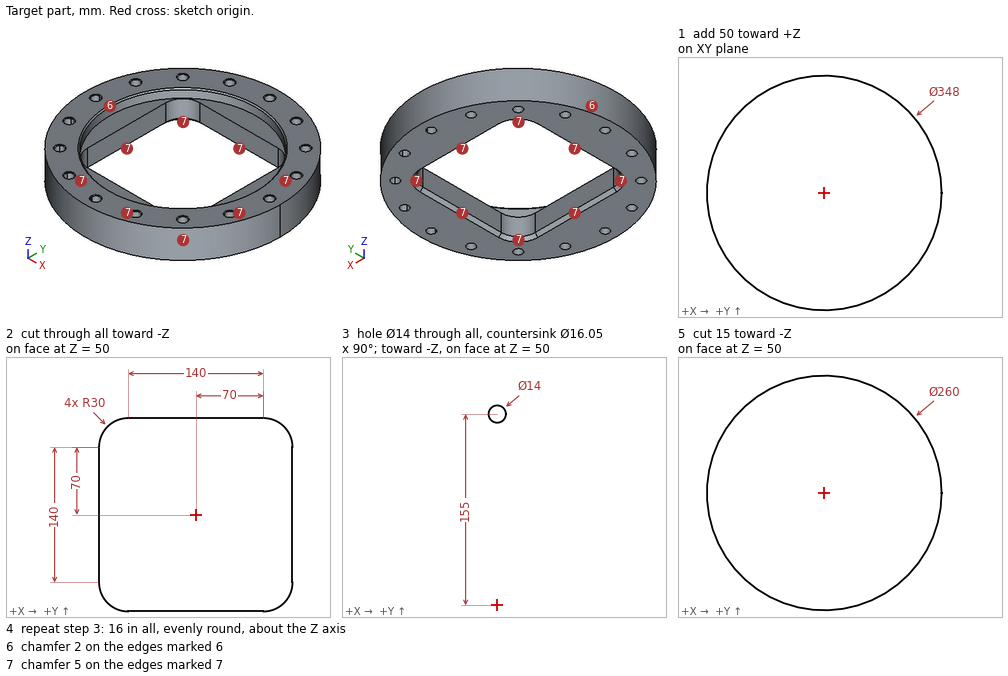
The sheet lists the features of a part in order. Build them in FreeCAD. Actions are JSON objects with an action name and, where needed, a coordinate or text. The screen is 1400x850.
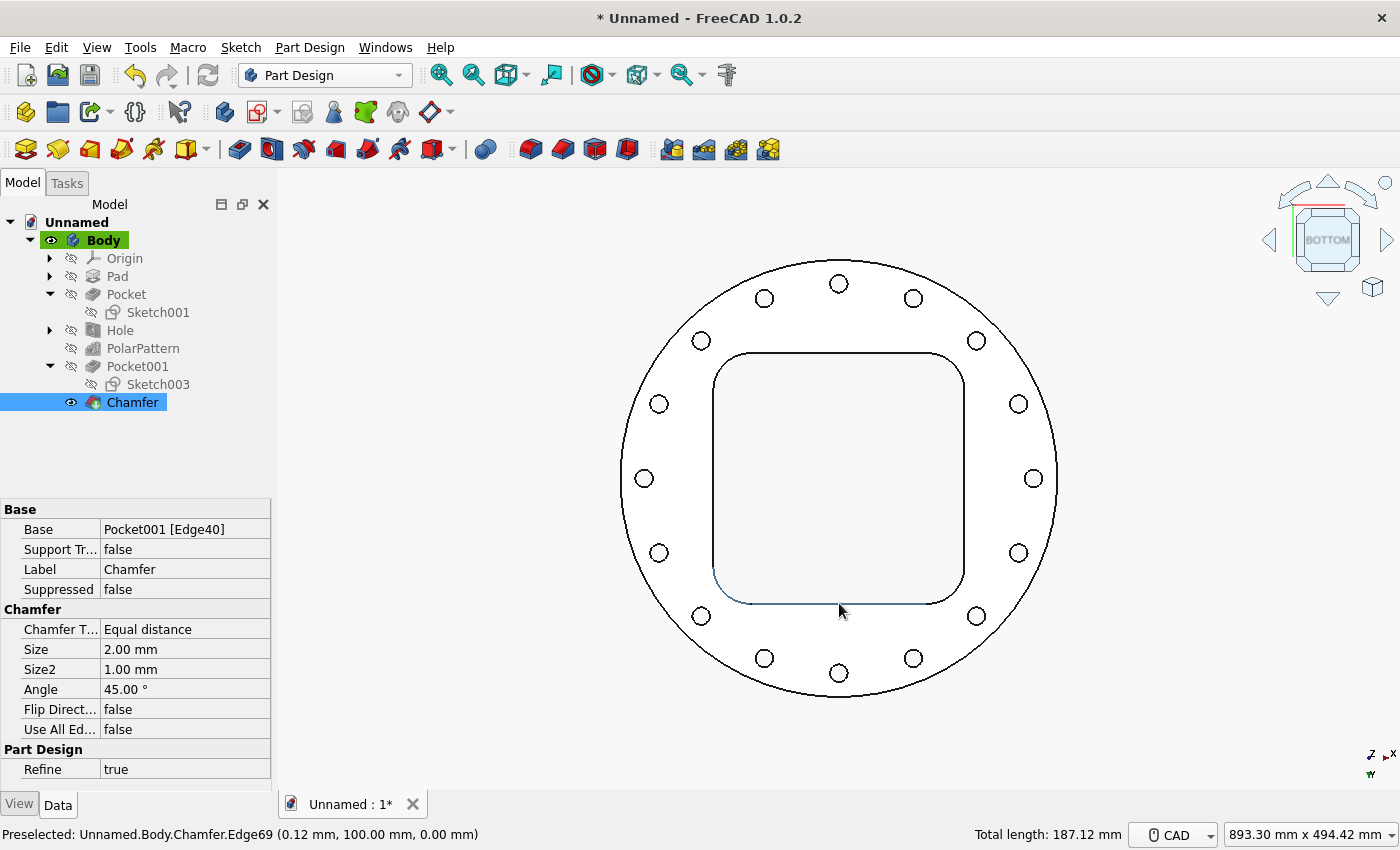
{"action": "left_click", "coordinate": [953, 592], "text": "ctrl"}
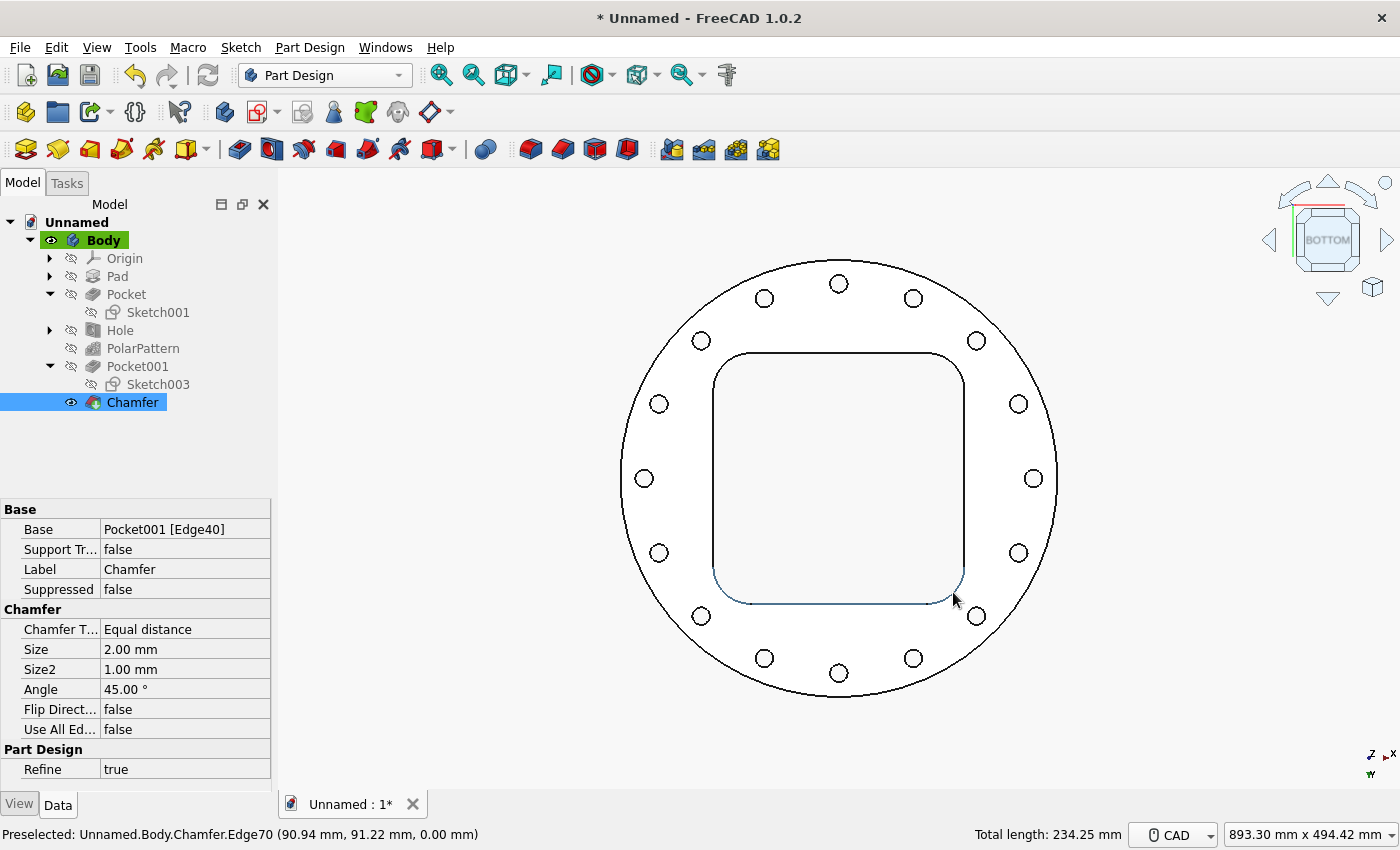
{"action": "left_click", "coordinate": [964, 477], "text": "ctrl"}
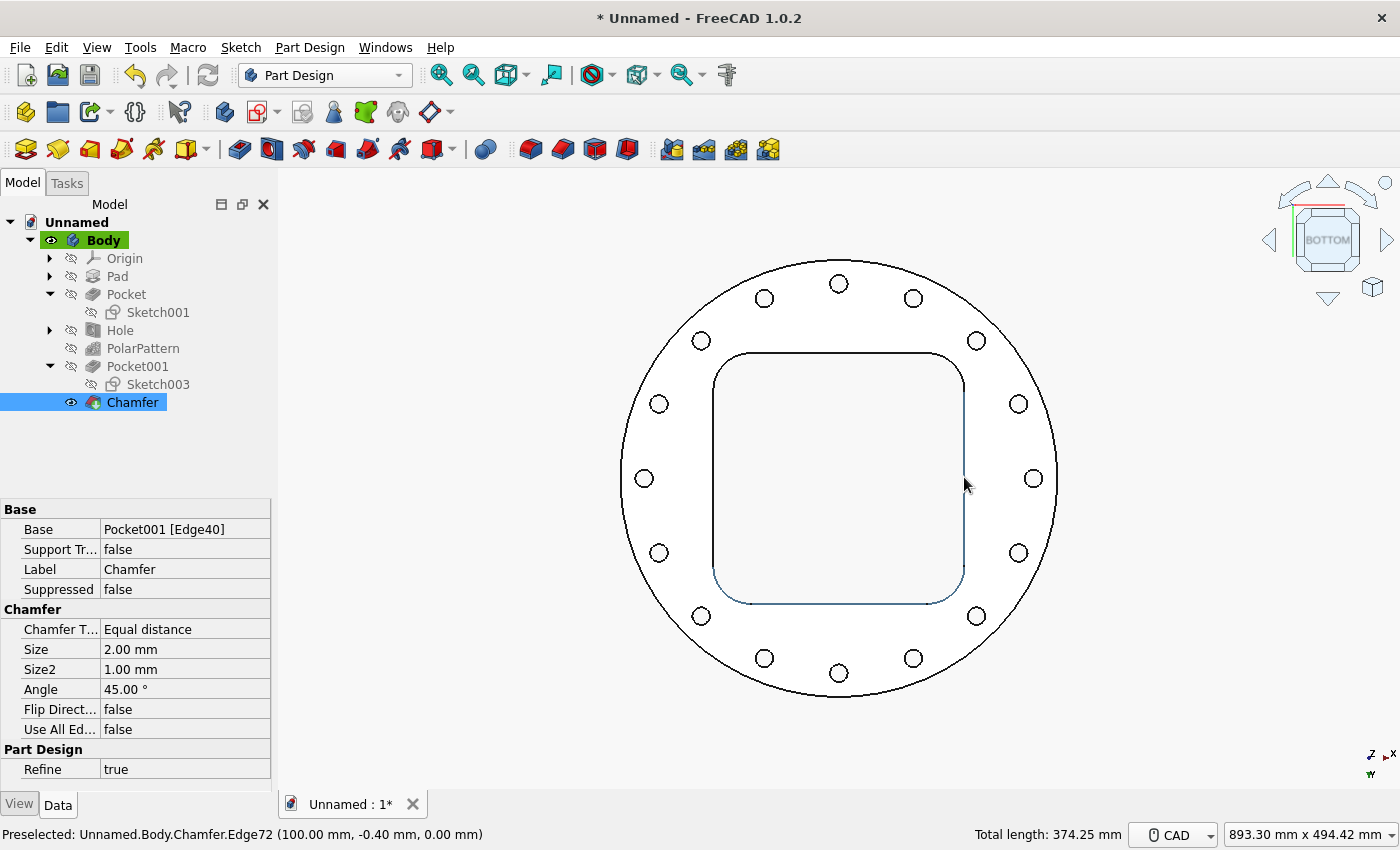
{"action": "left_click", "coordinate": [949, 359], "text": "ctrl"}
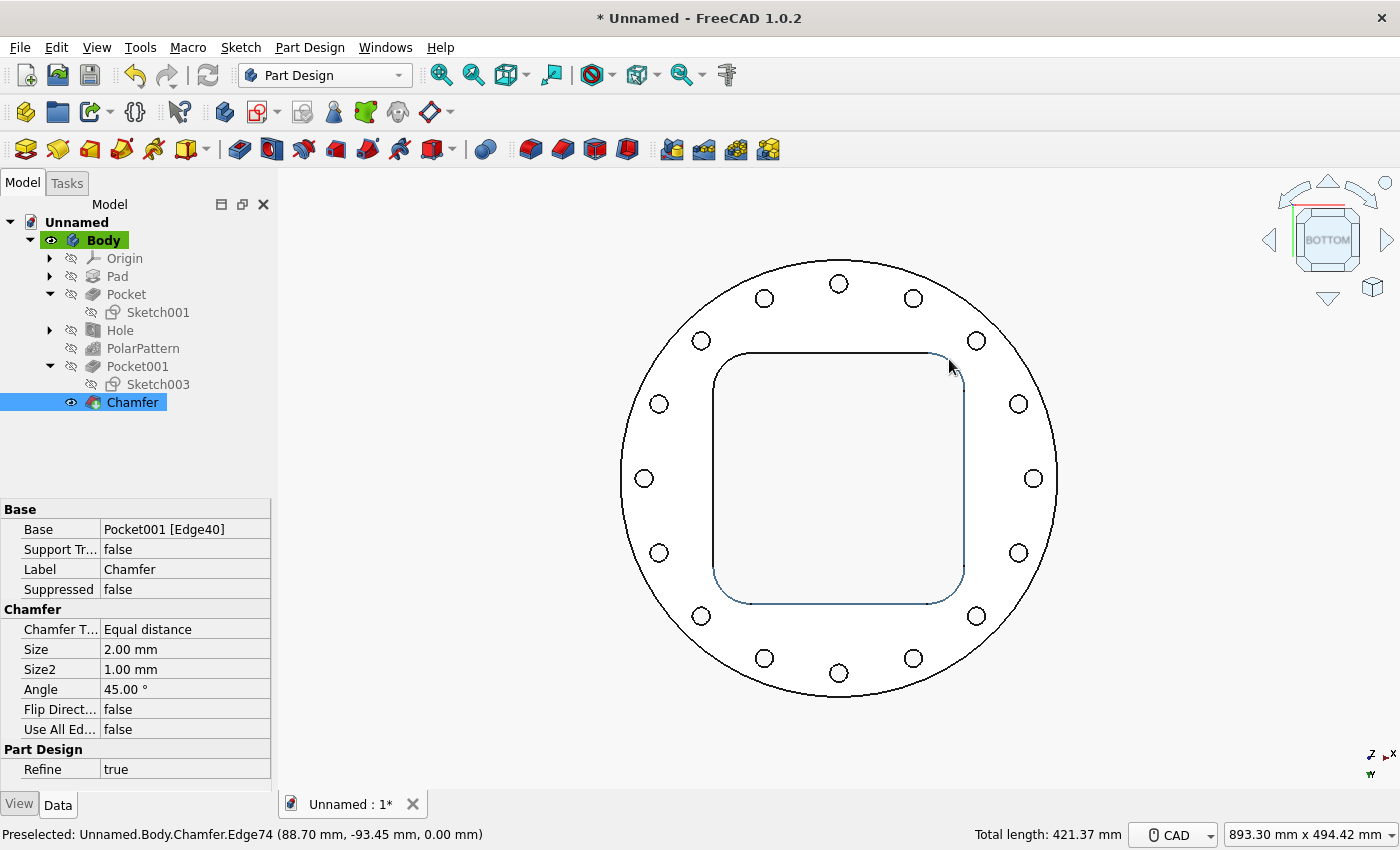
{"action": "key", "text": "4"}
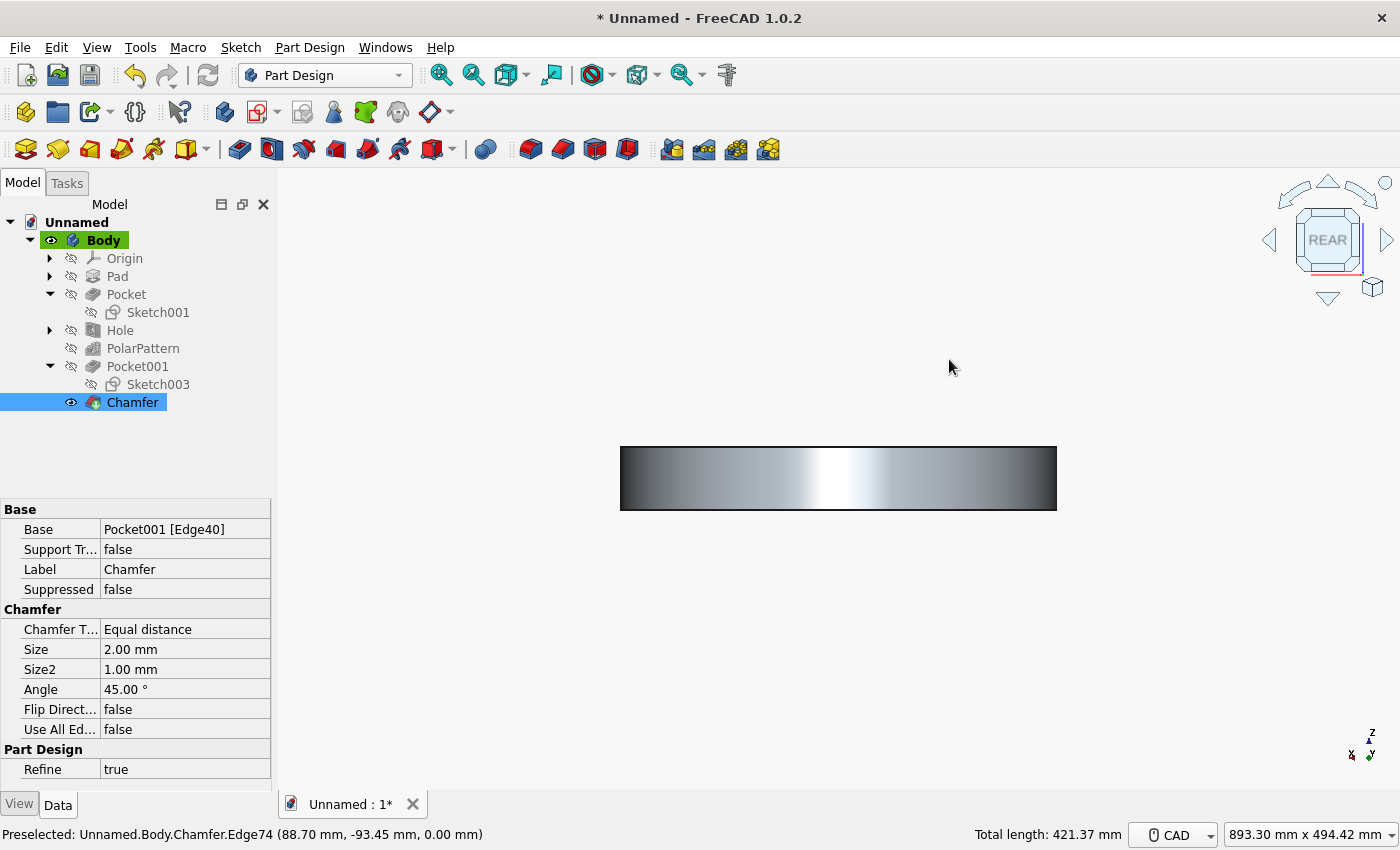
{"action": "left_click", "coordinate": [442, 76]}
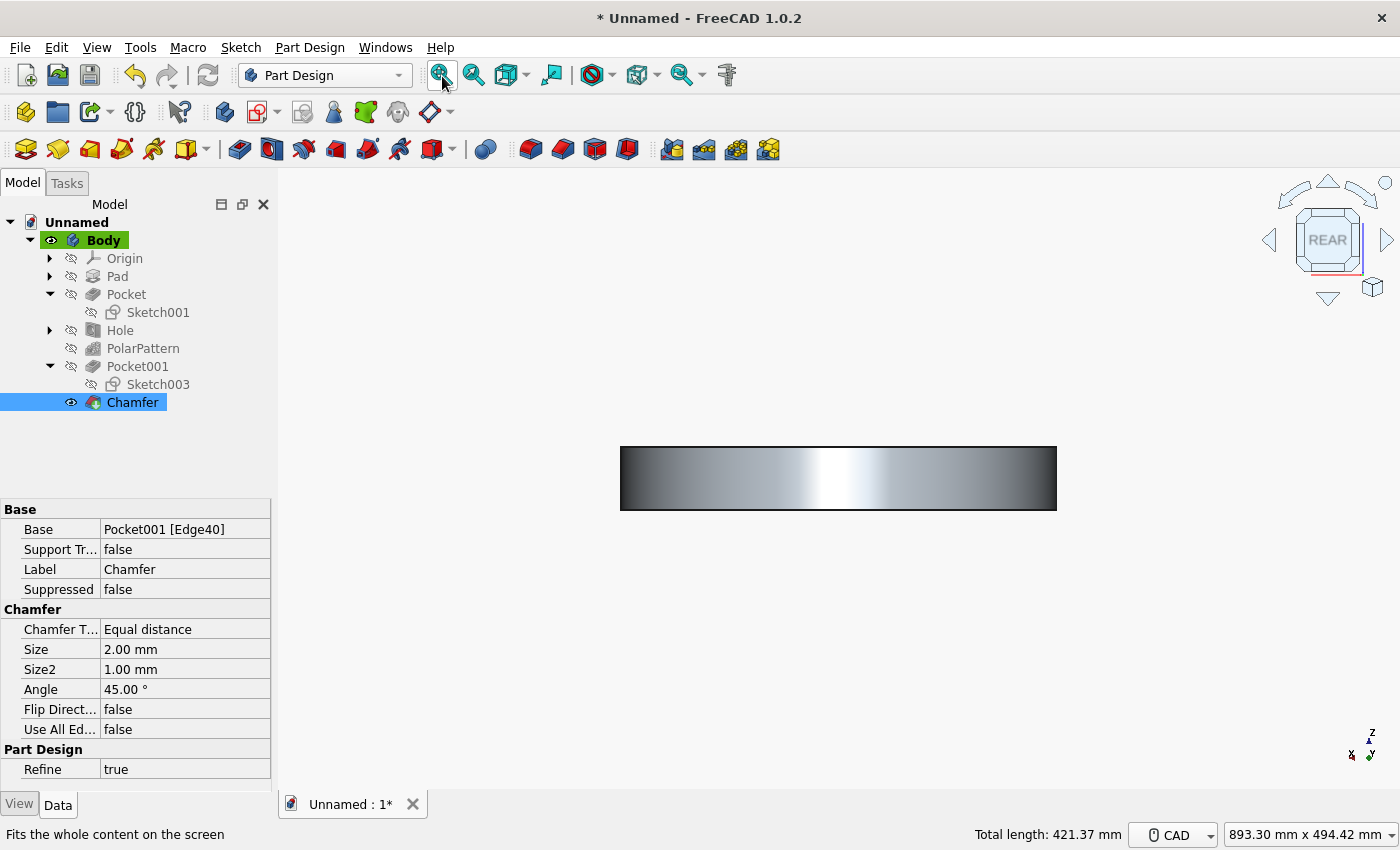
{"action": "key", "text": "6"}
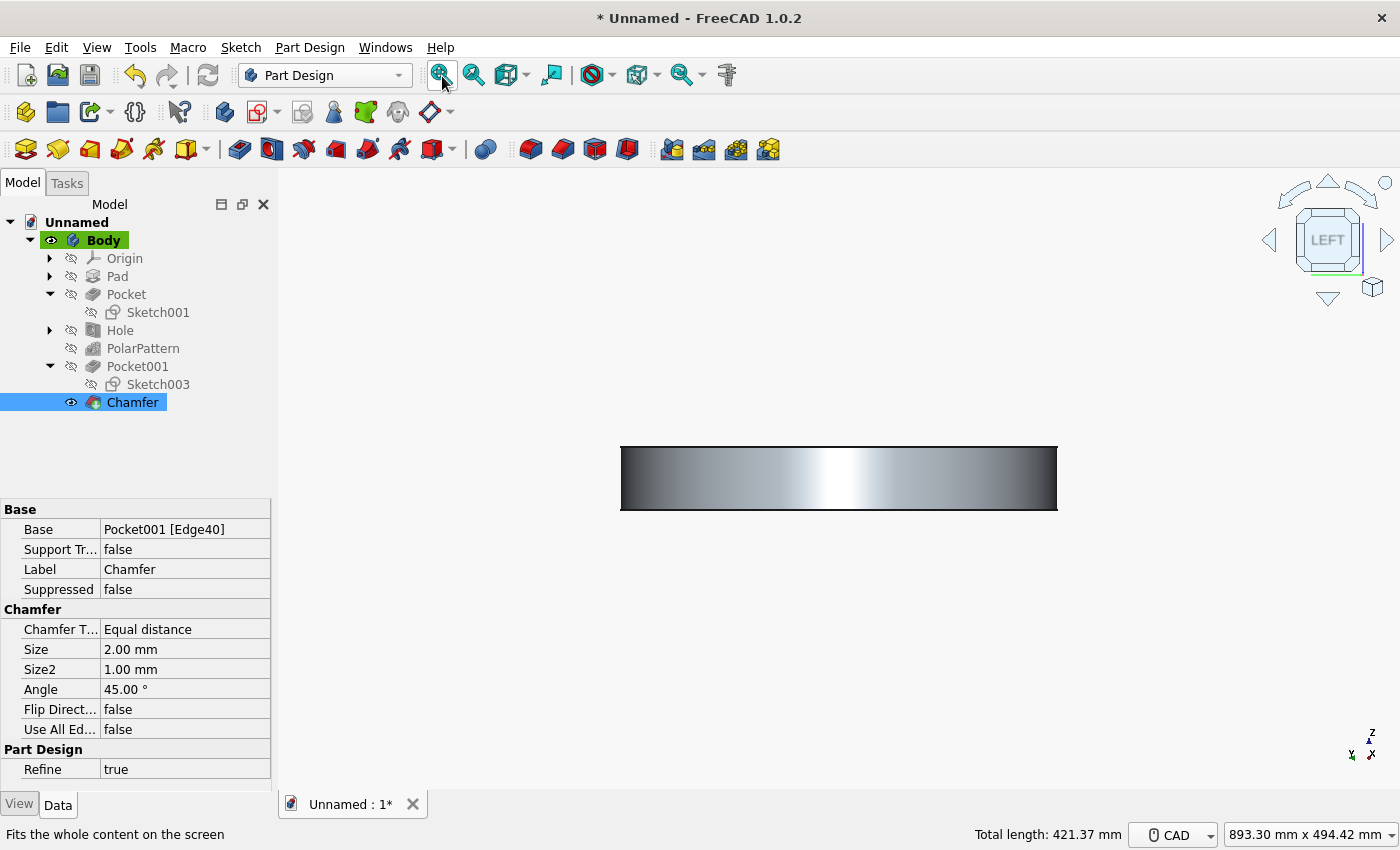
{"action": "left_click", "coordinate": [442, 76]}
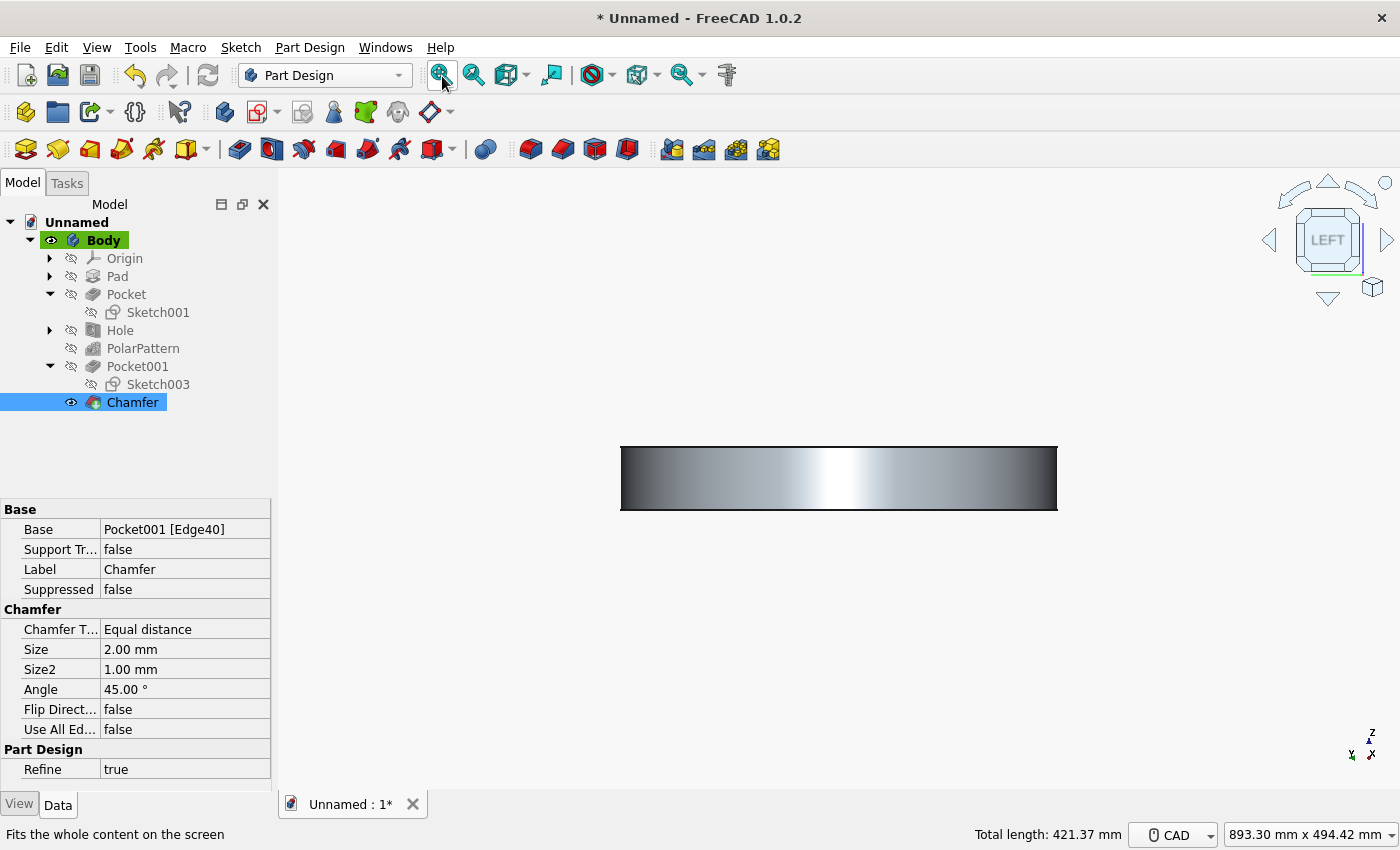
{"action": "key", "text": "v 3"}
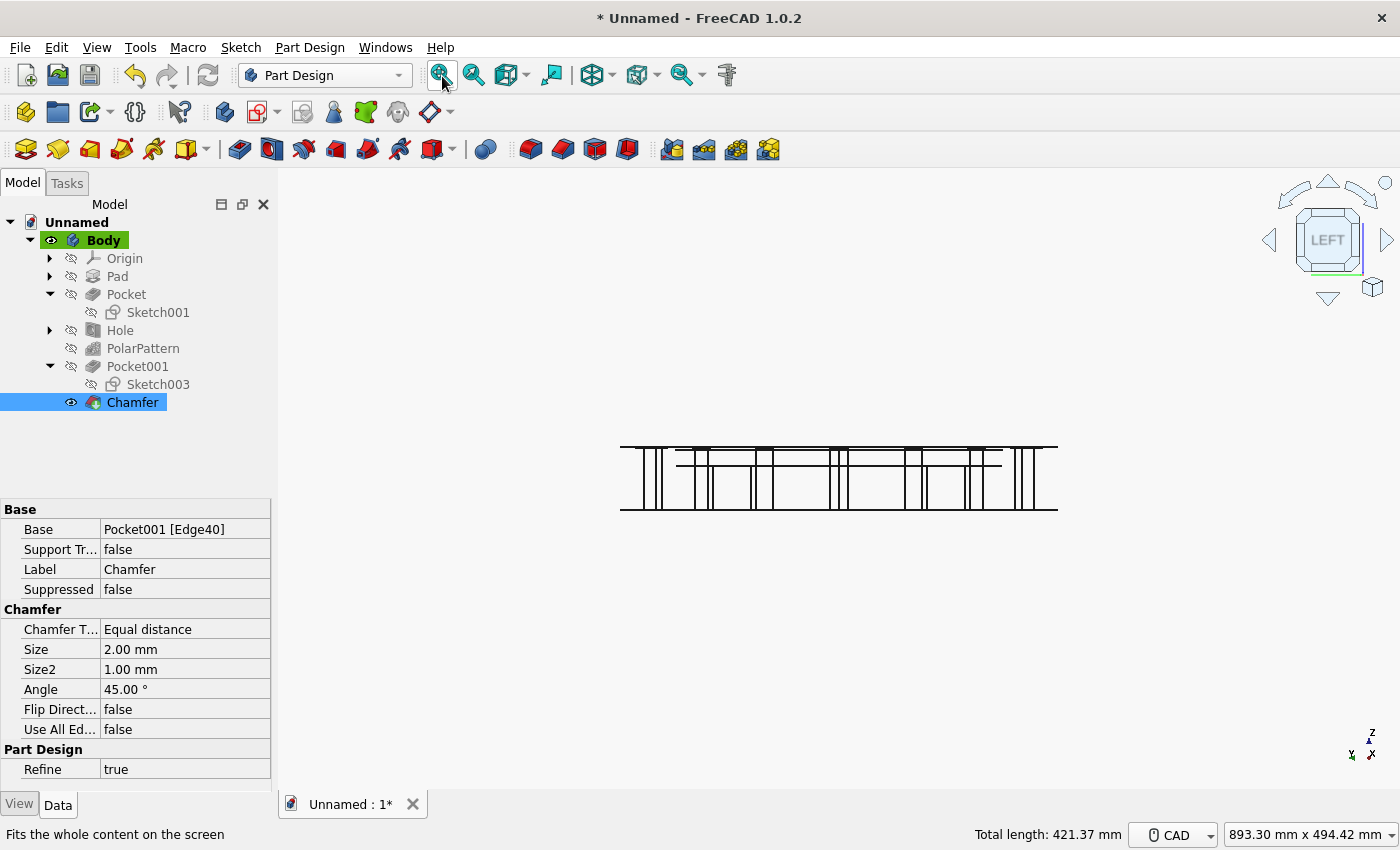
{"action": "key", "text": "0"}